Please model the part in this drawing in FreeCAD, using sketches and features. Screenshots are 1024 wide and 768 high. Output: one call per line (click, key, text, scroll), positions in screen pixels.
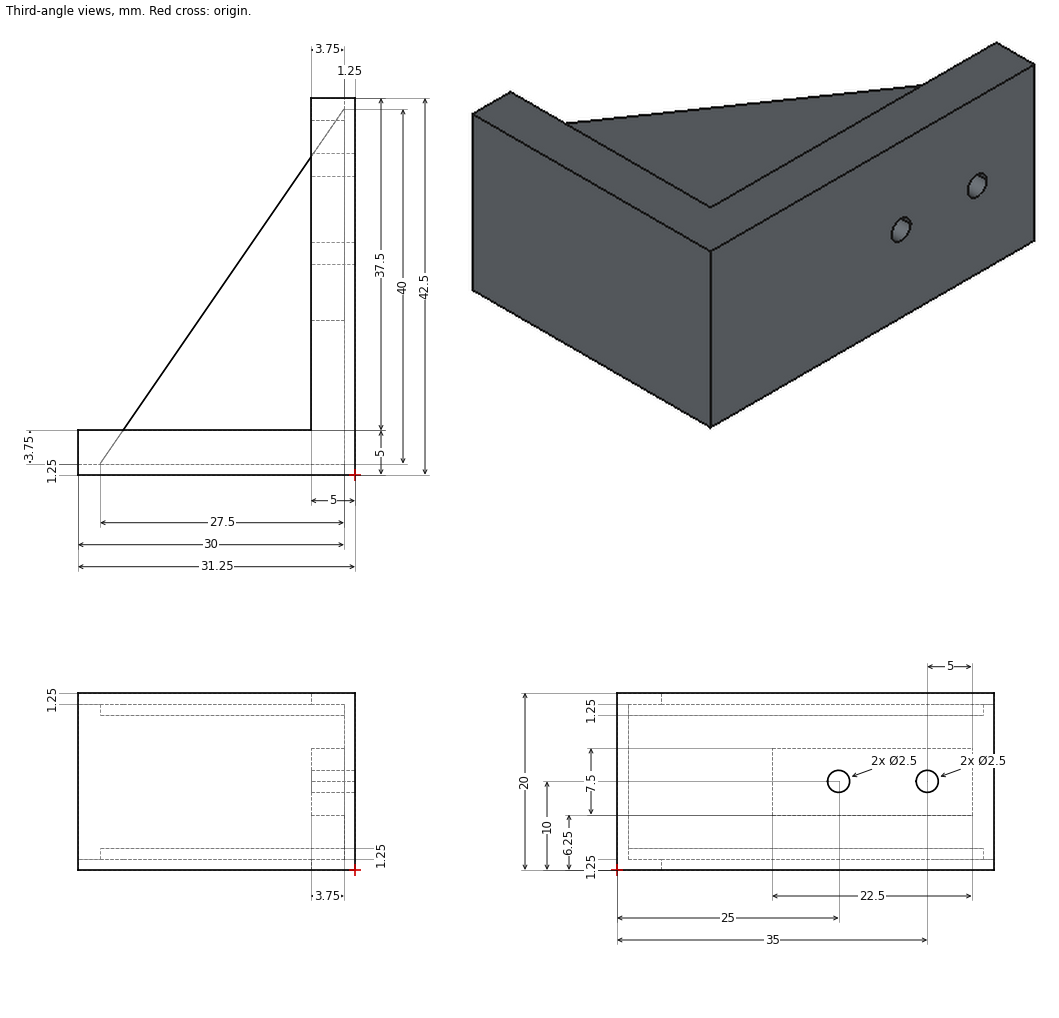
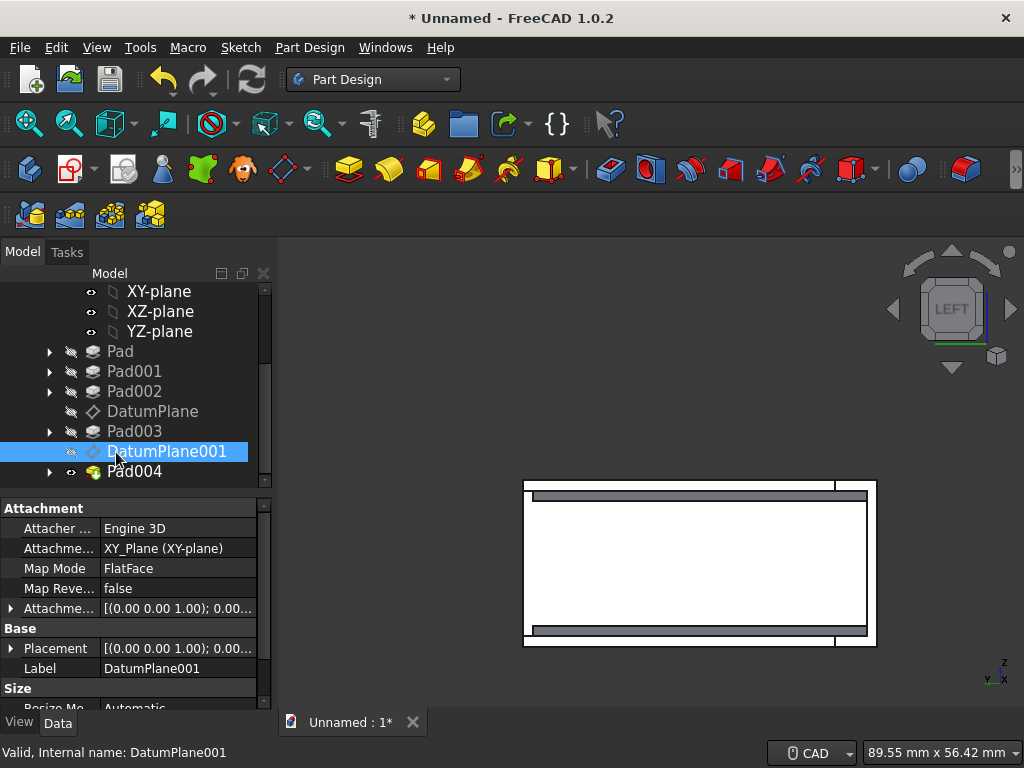
click(597, 562)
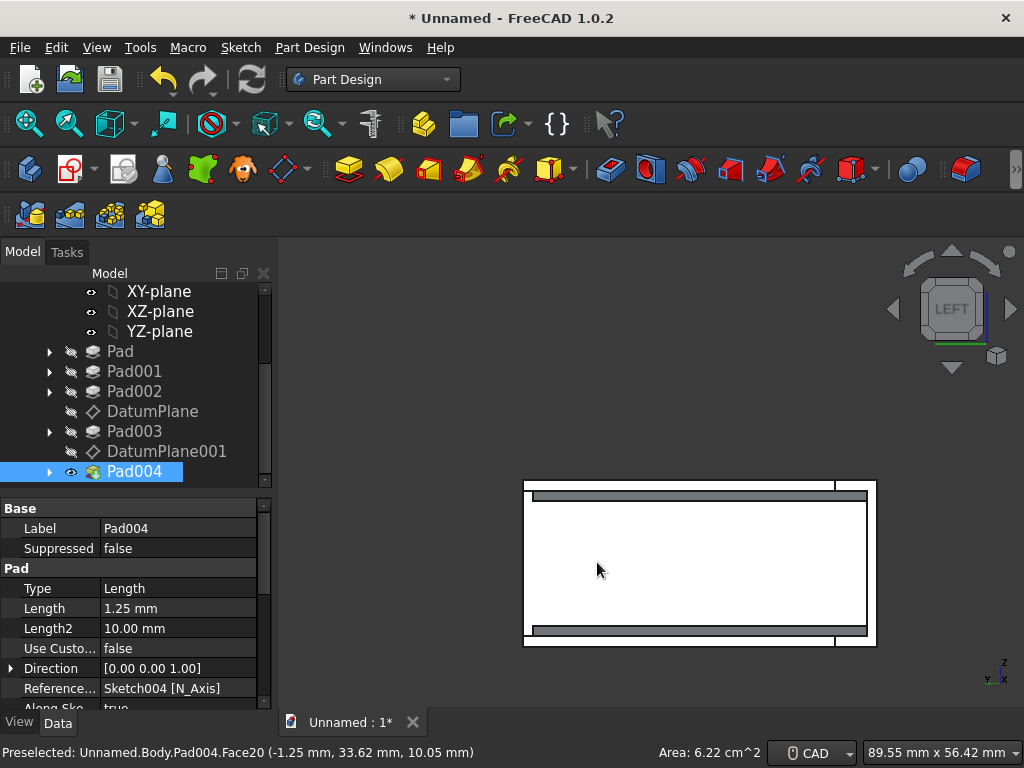
click(70, 170)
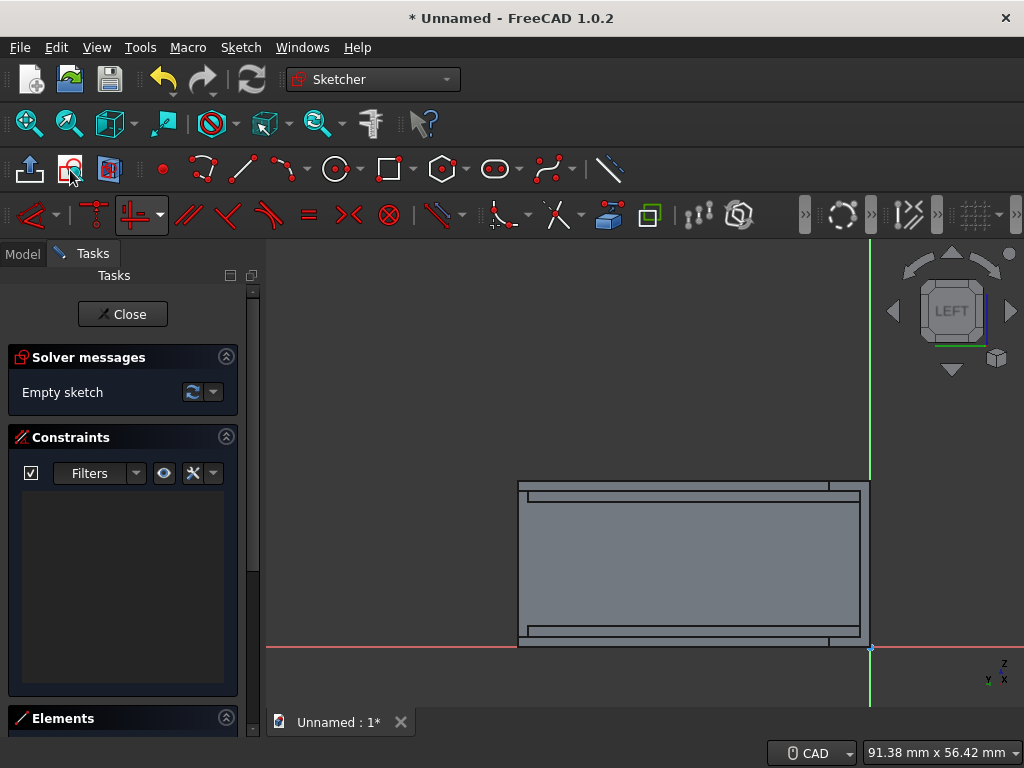
click(110, 170)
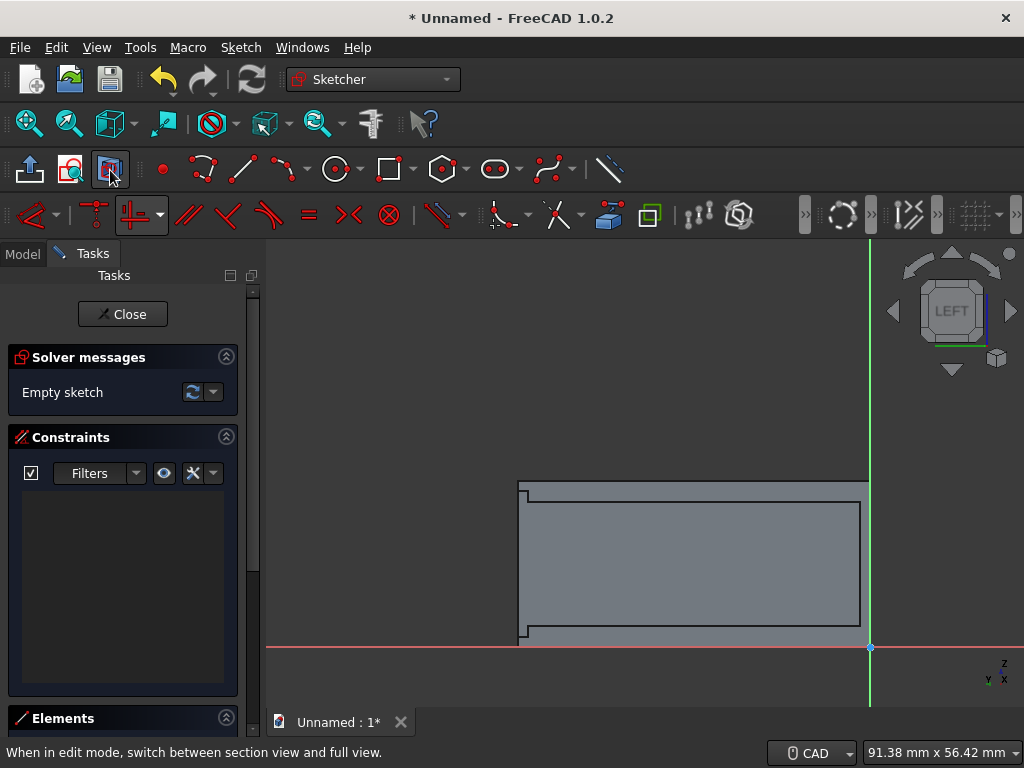
scroll(294, 267, down, 1)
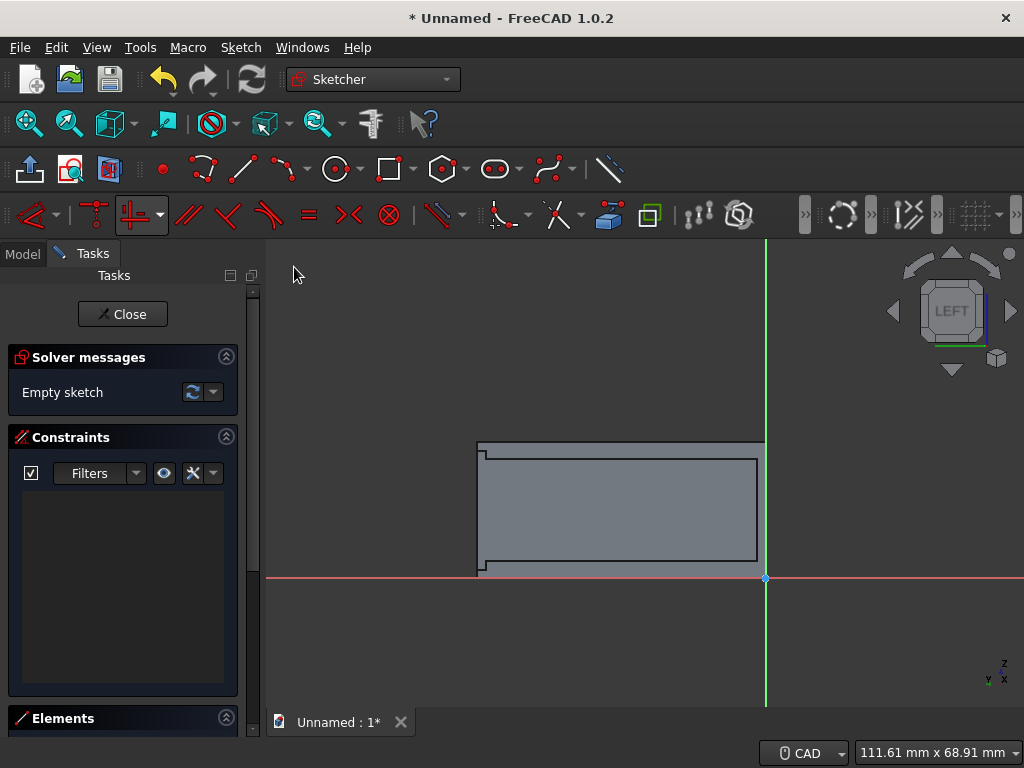
scroll(738, 650, up, 2)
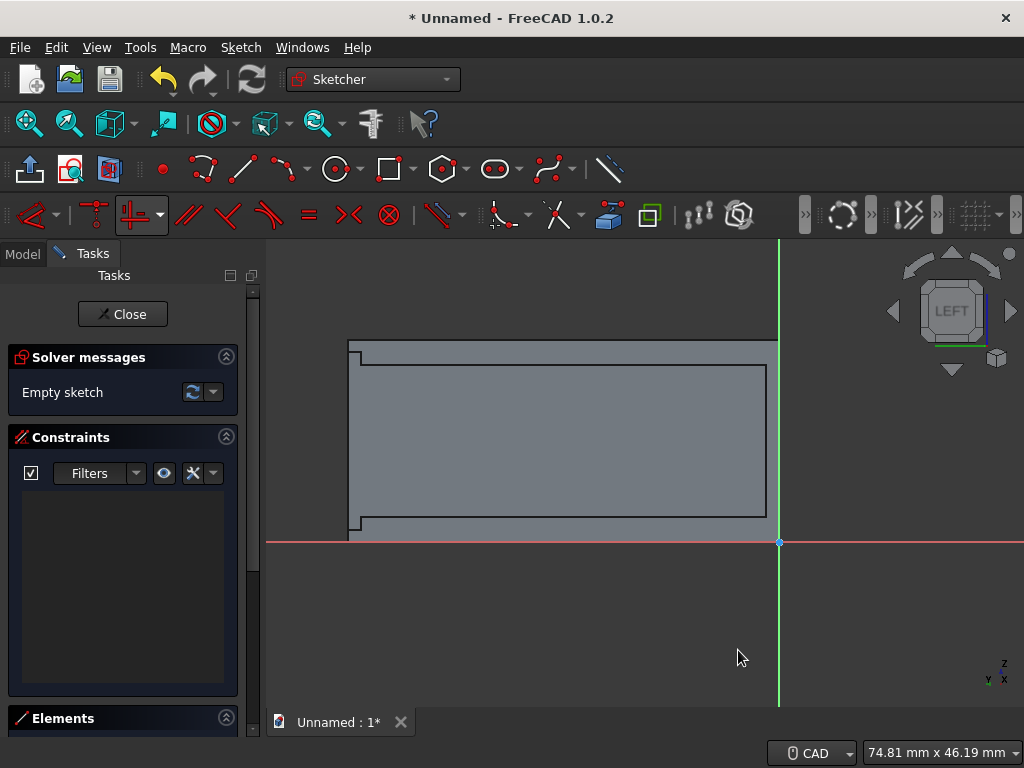
click(390, 170)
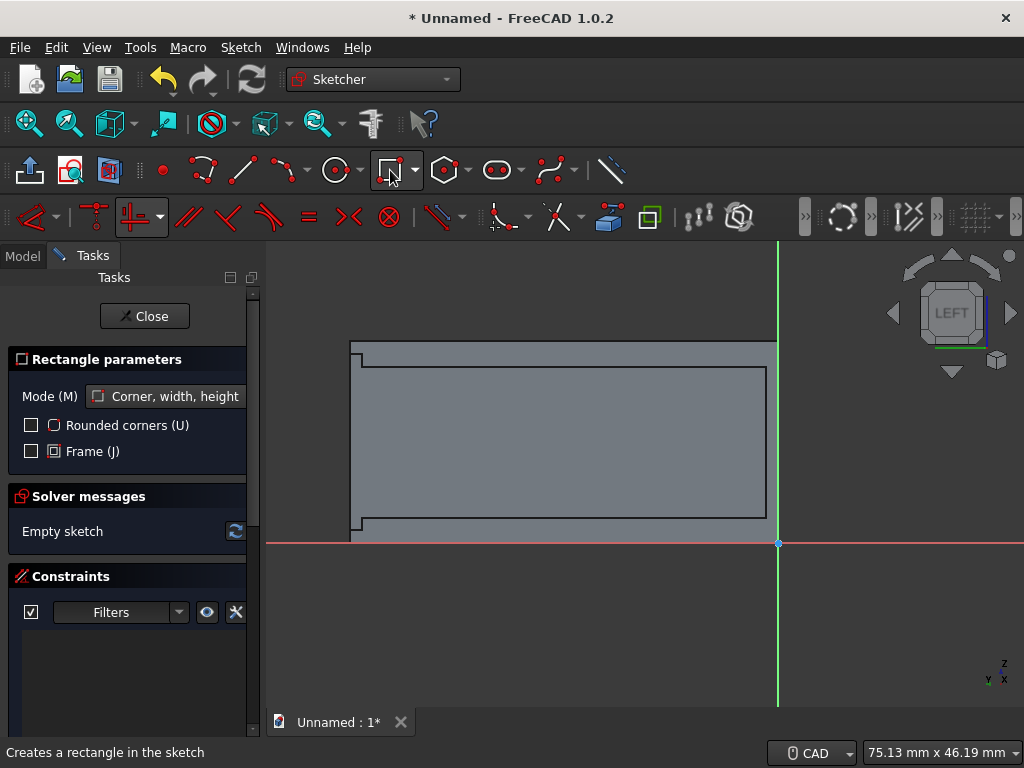
click(375, 404)
move(602, 480)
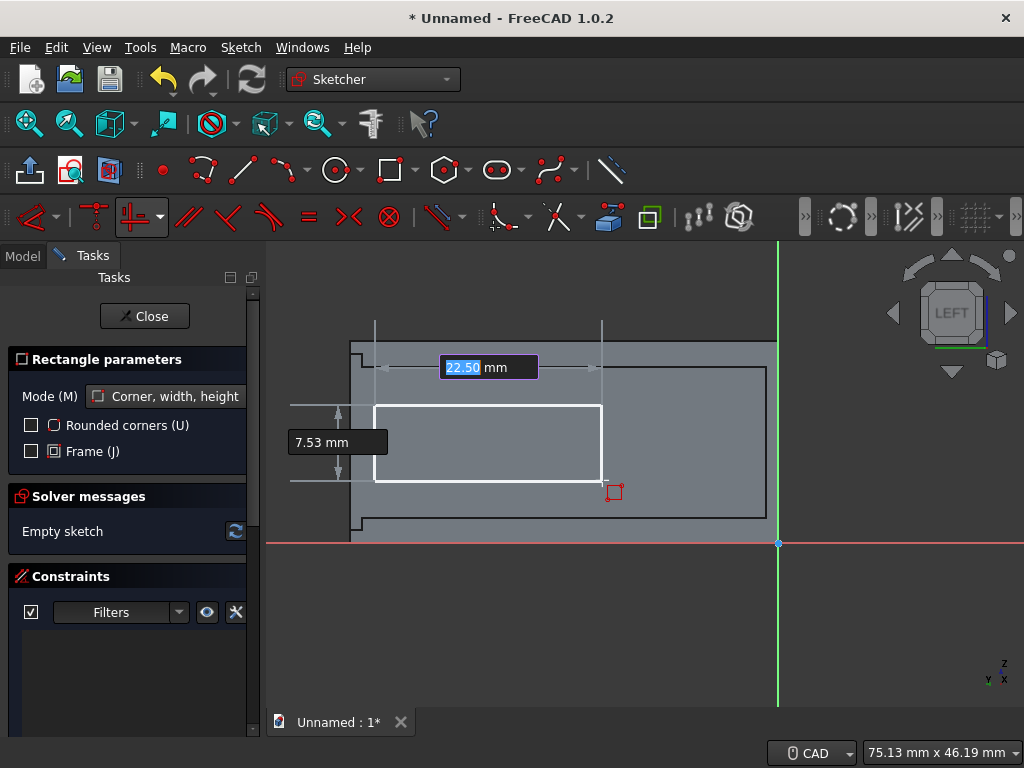
text(22.5)
key(Tab)
text(7.5)
key(Return)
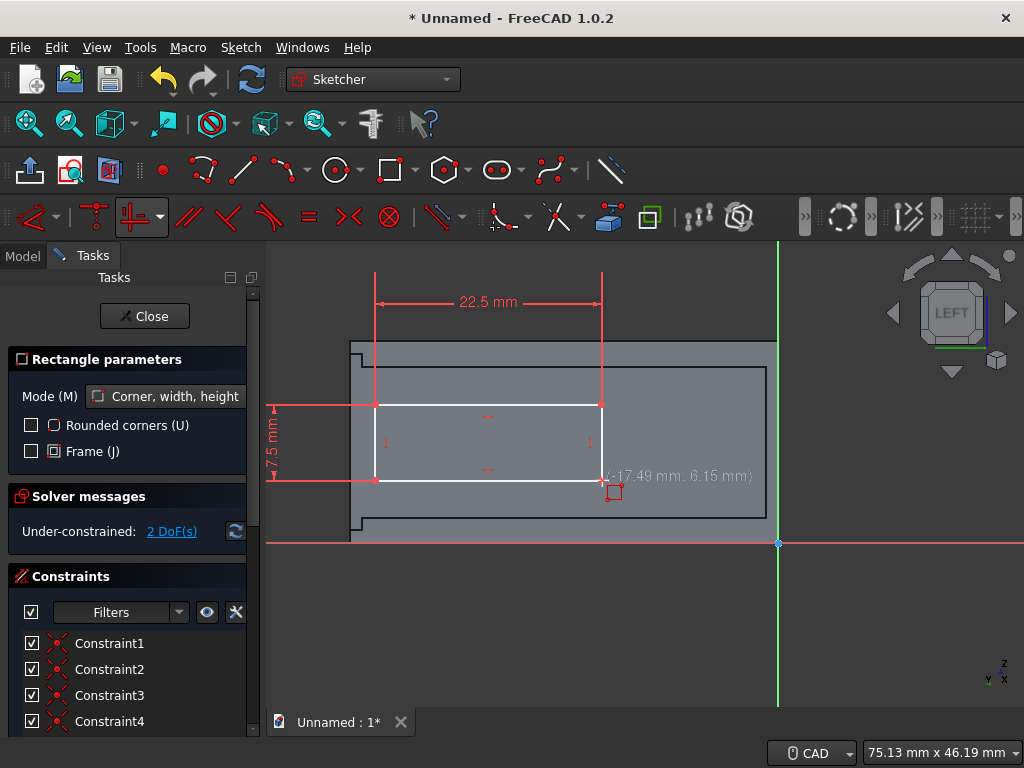
key(g)
key(c)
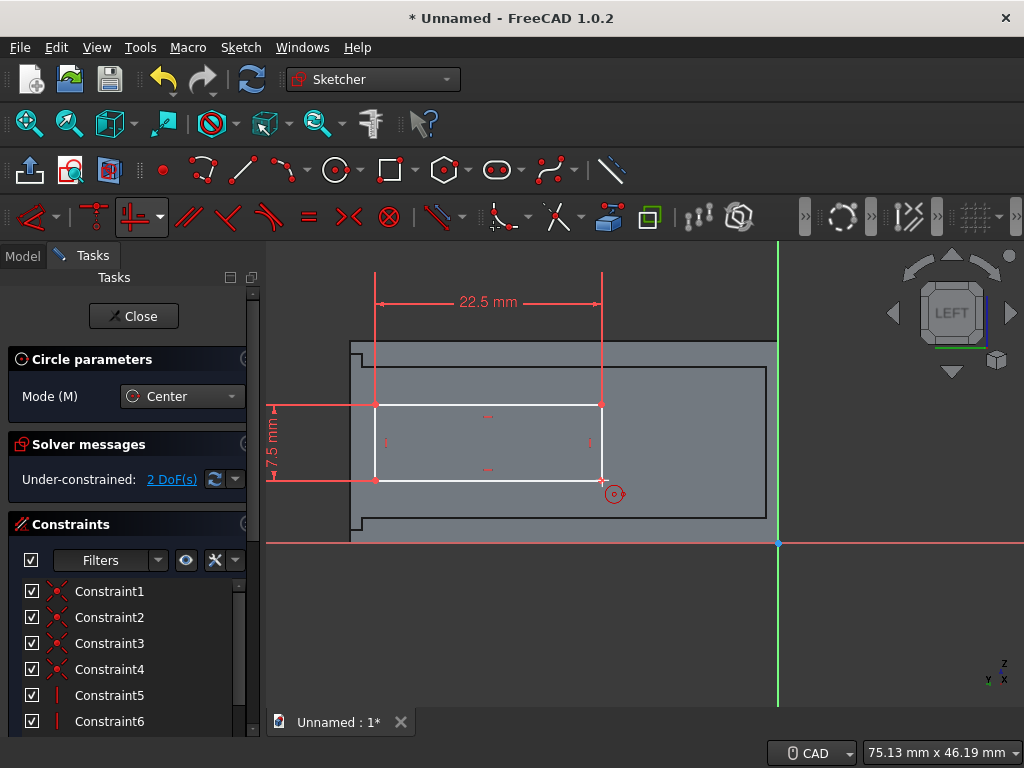
scroll(526, 442, up, 3)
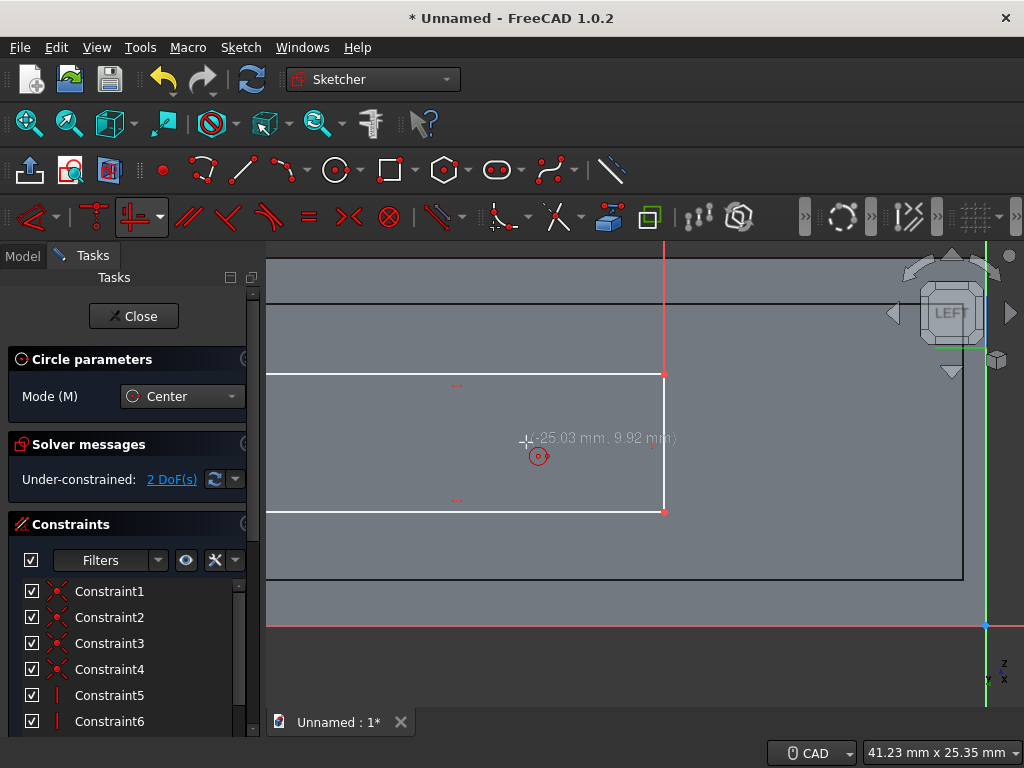
click(526, 442)
move(542, 426)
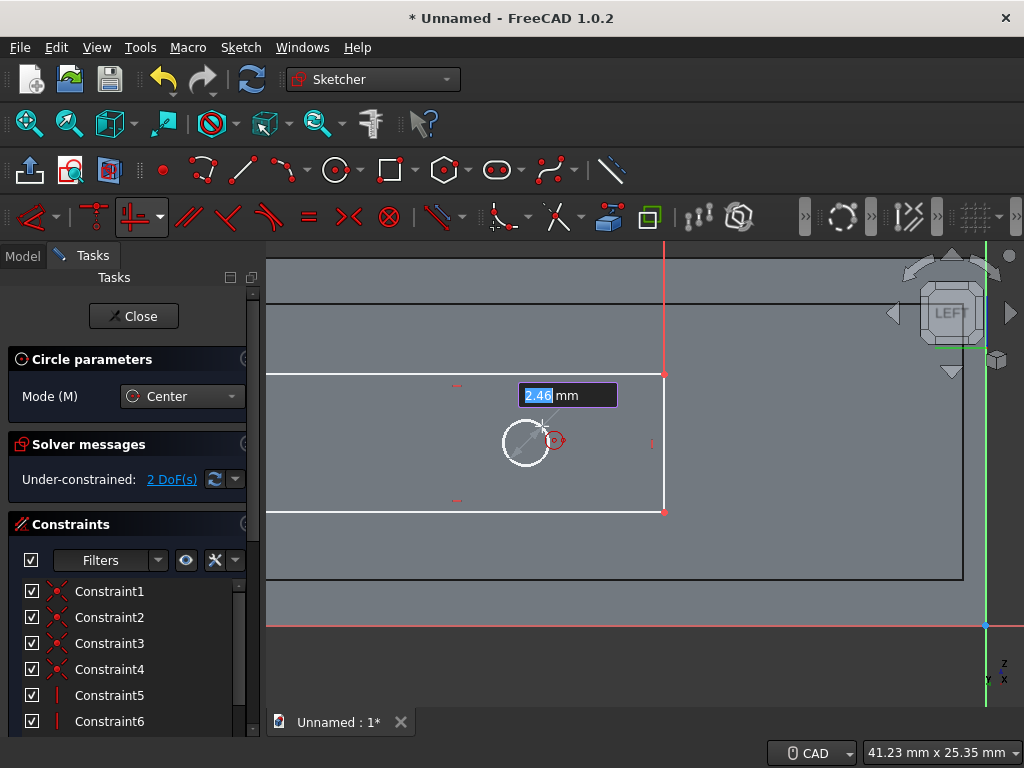
text(2.5)
key(Return)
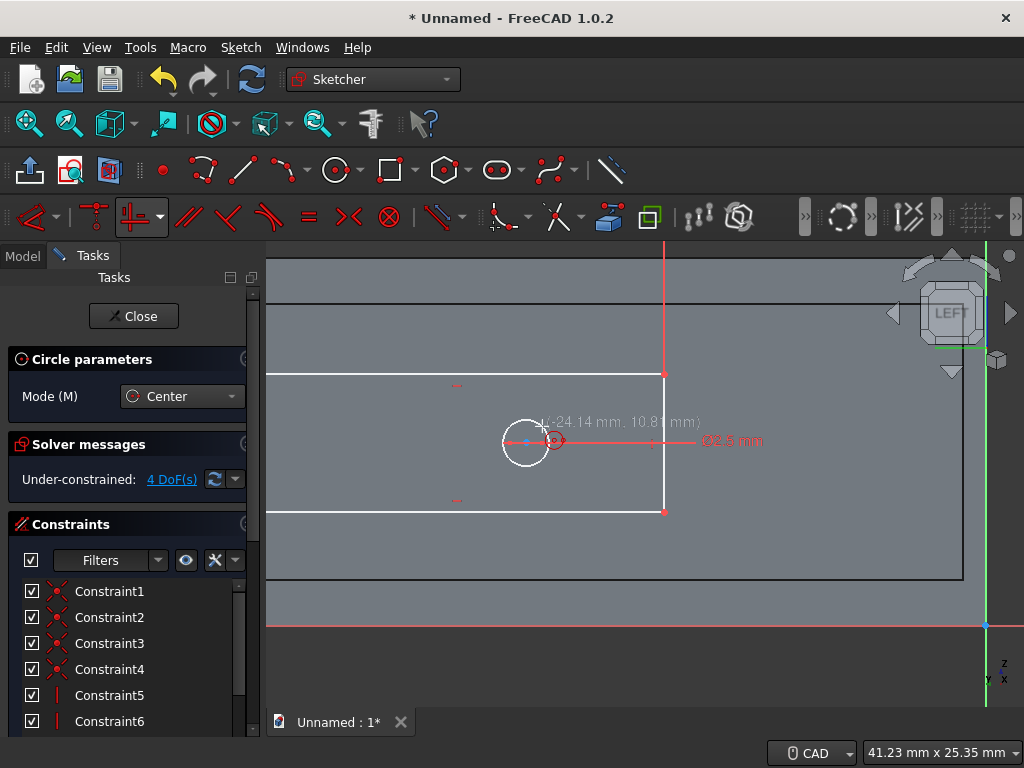
click(342, 442)
move(359, 426)